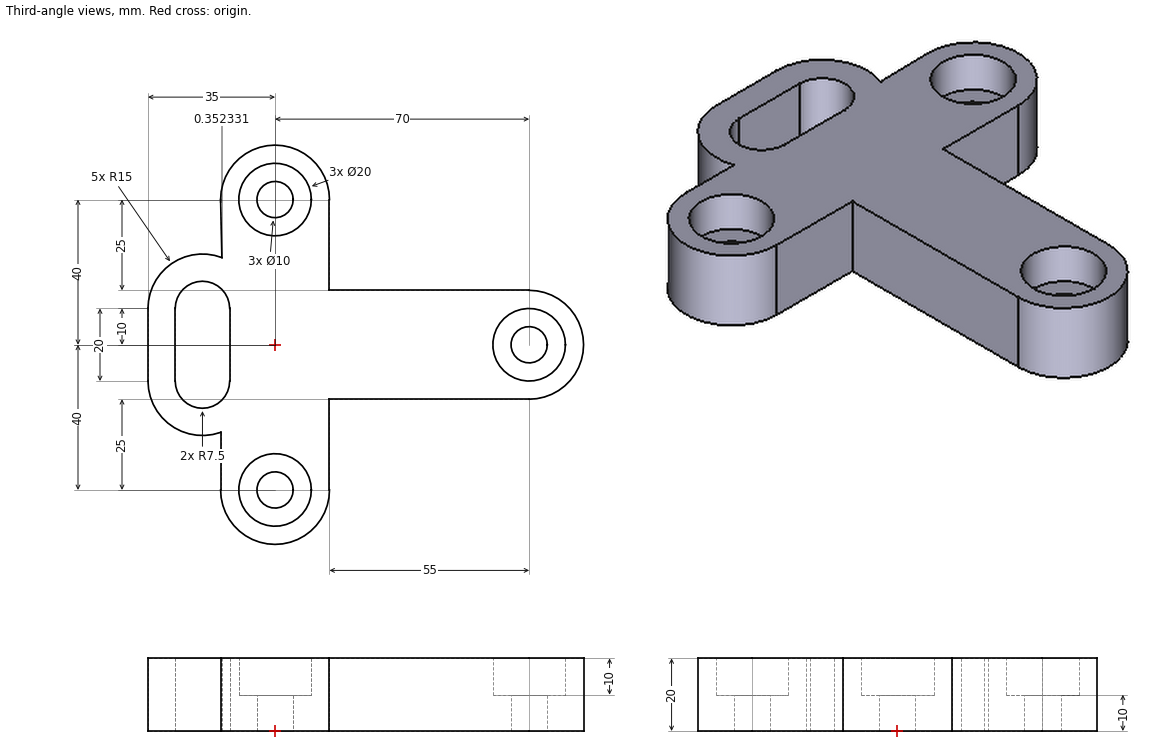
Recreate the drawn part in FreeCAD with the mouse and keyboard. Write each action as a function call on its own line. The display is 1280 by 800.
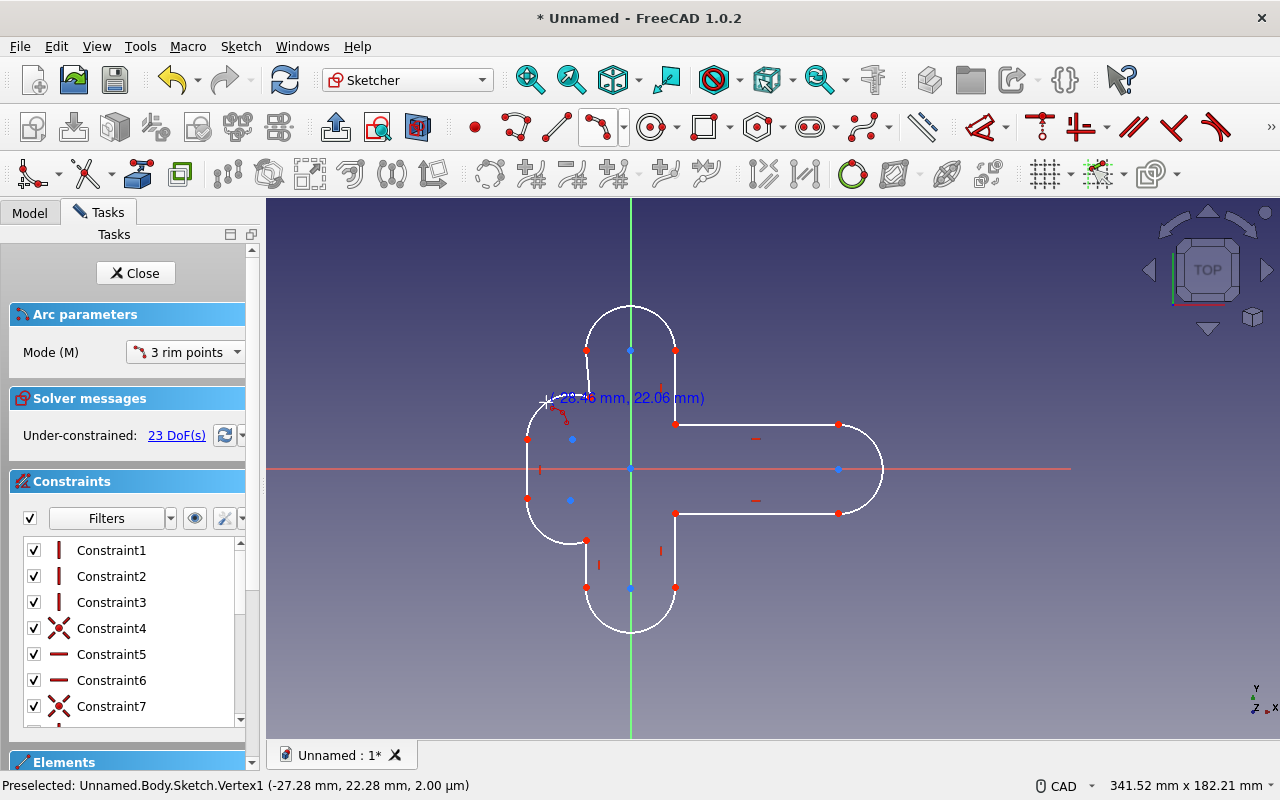
click(810, 128)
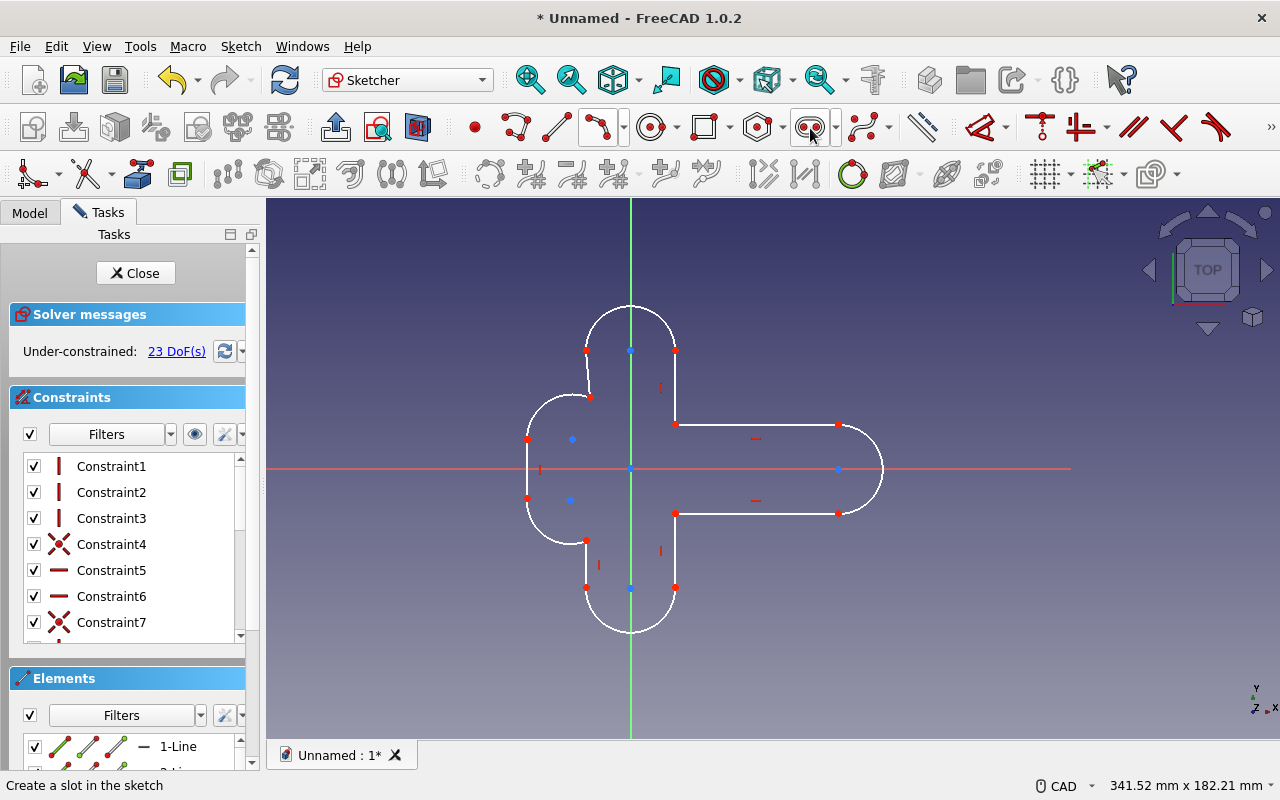
click(571, 498)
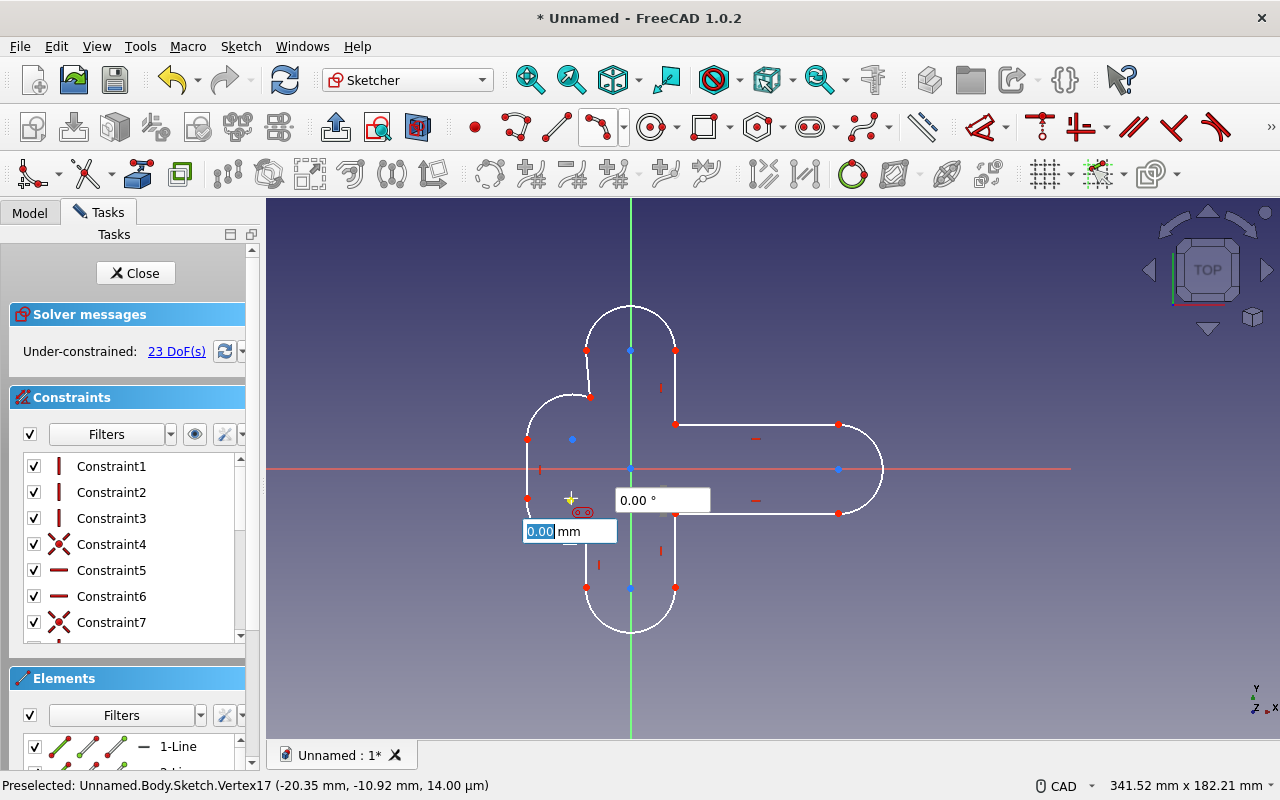
click(571, 439)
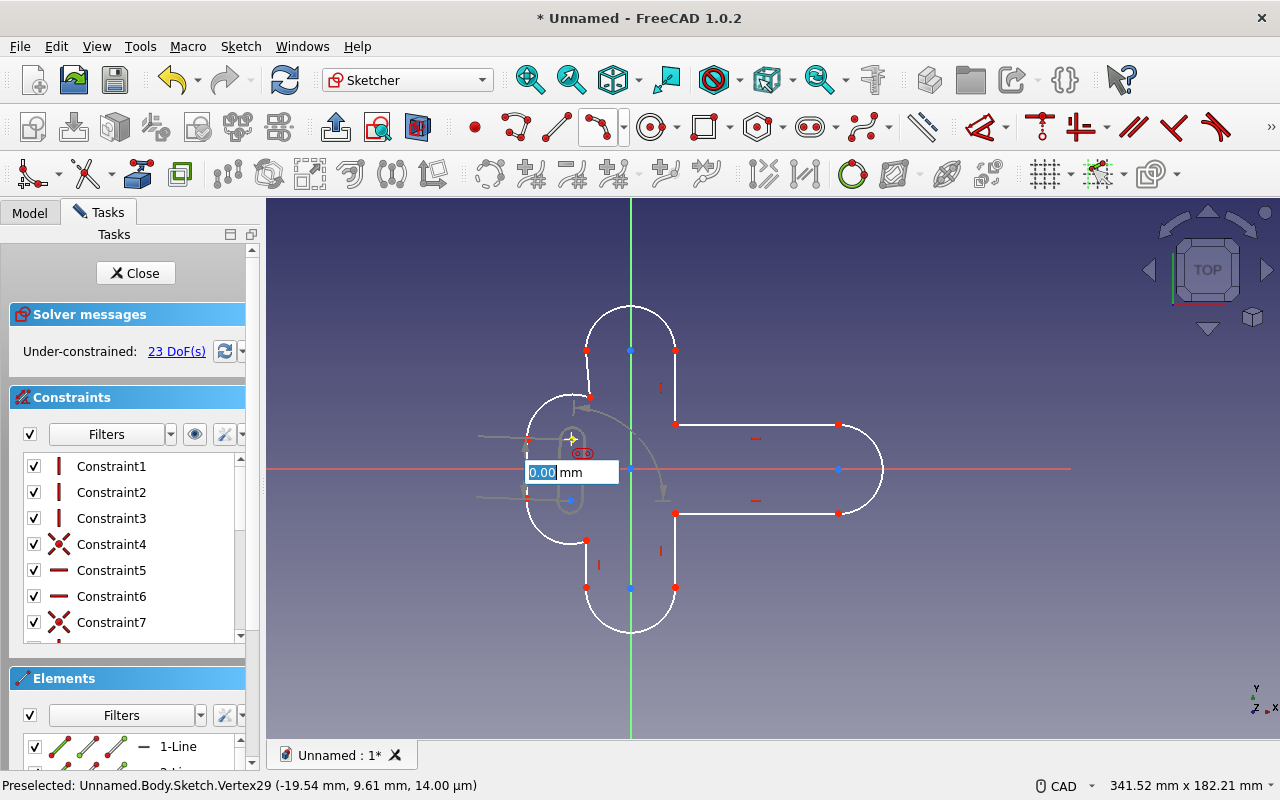
scroll(549, 477, up, 3)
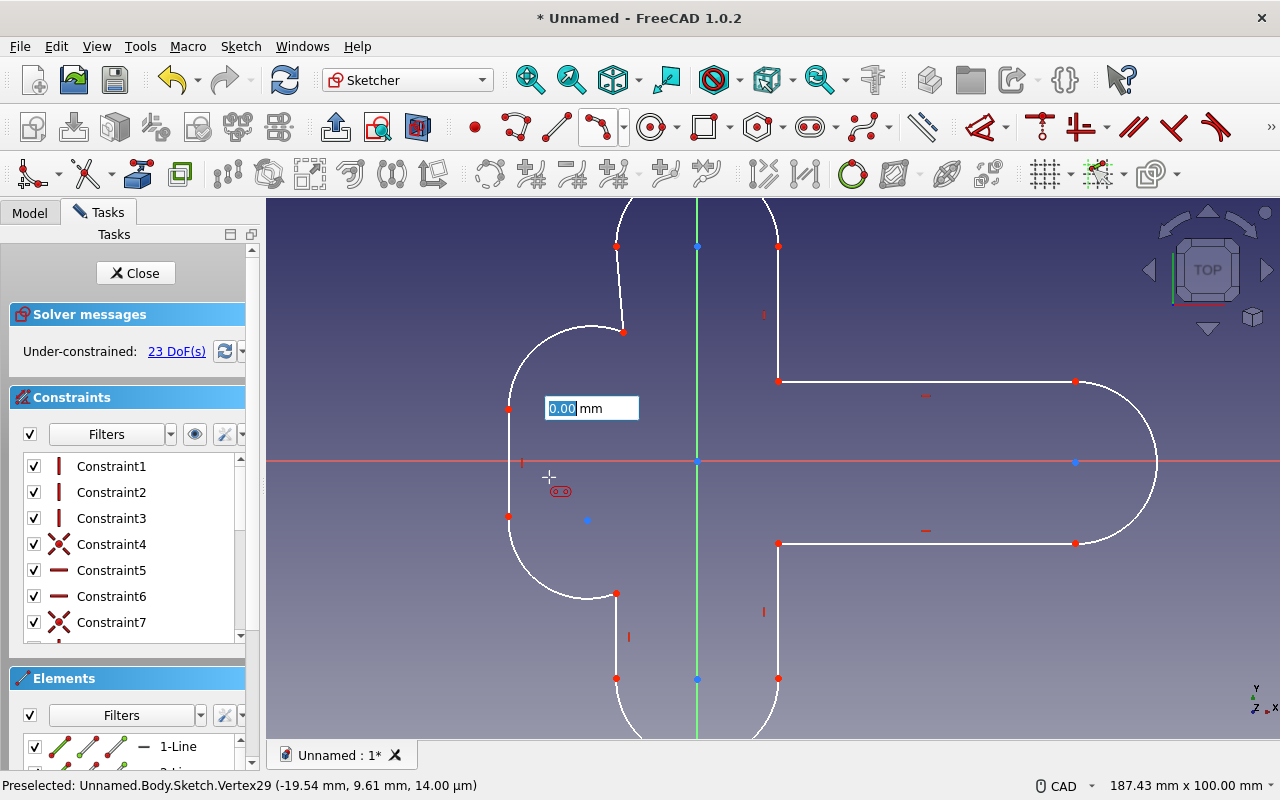
click(549, 477)
key(Escape)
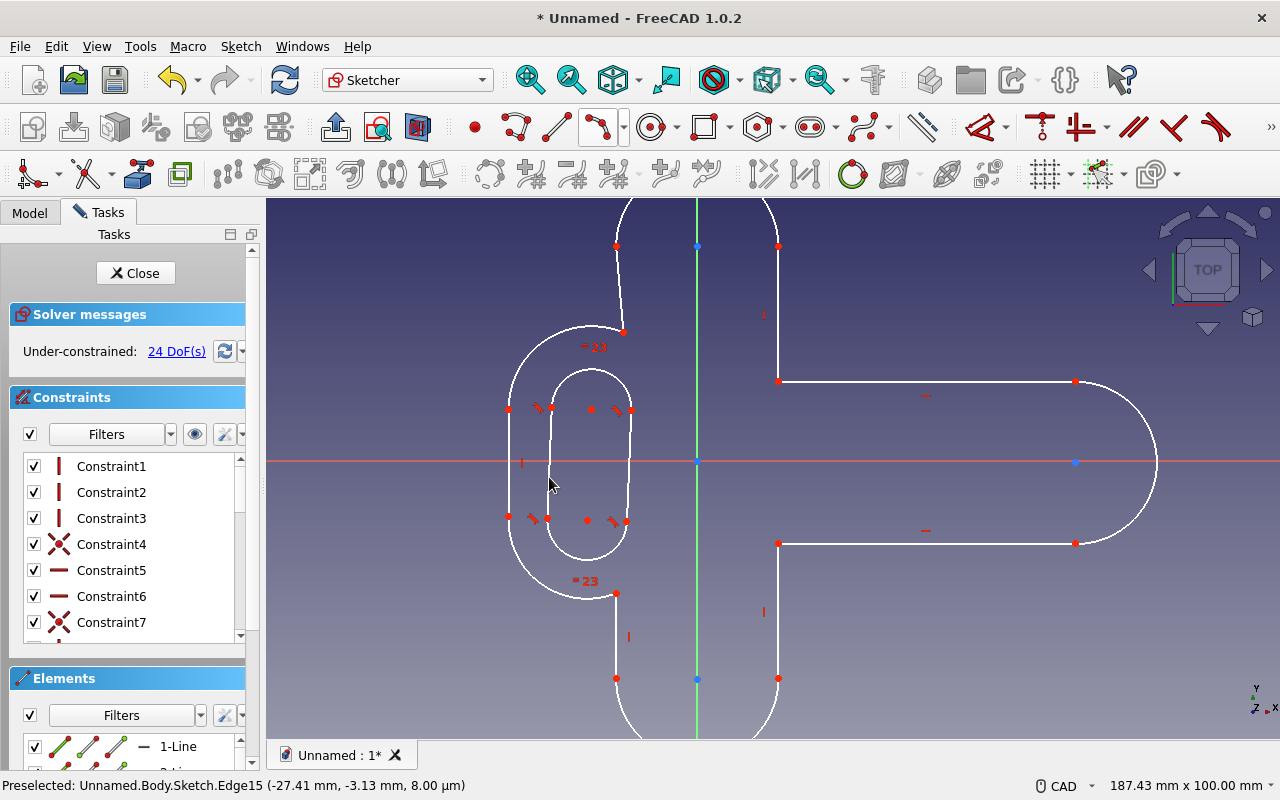
click(509, 441)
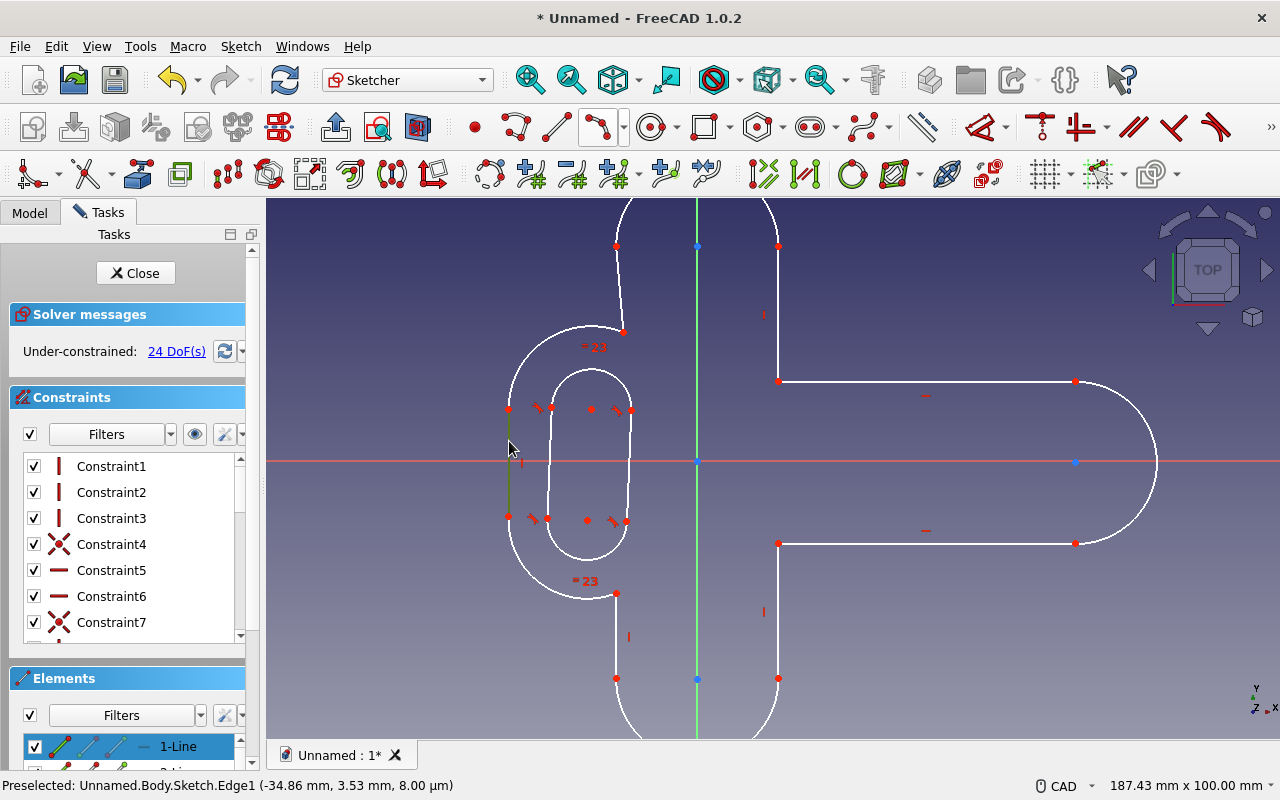
click(520, 561)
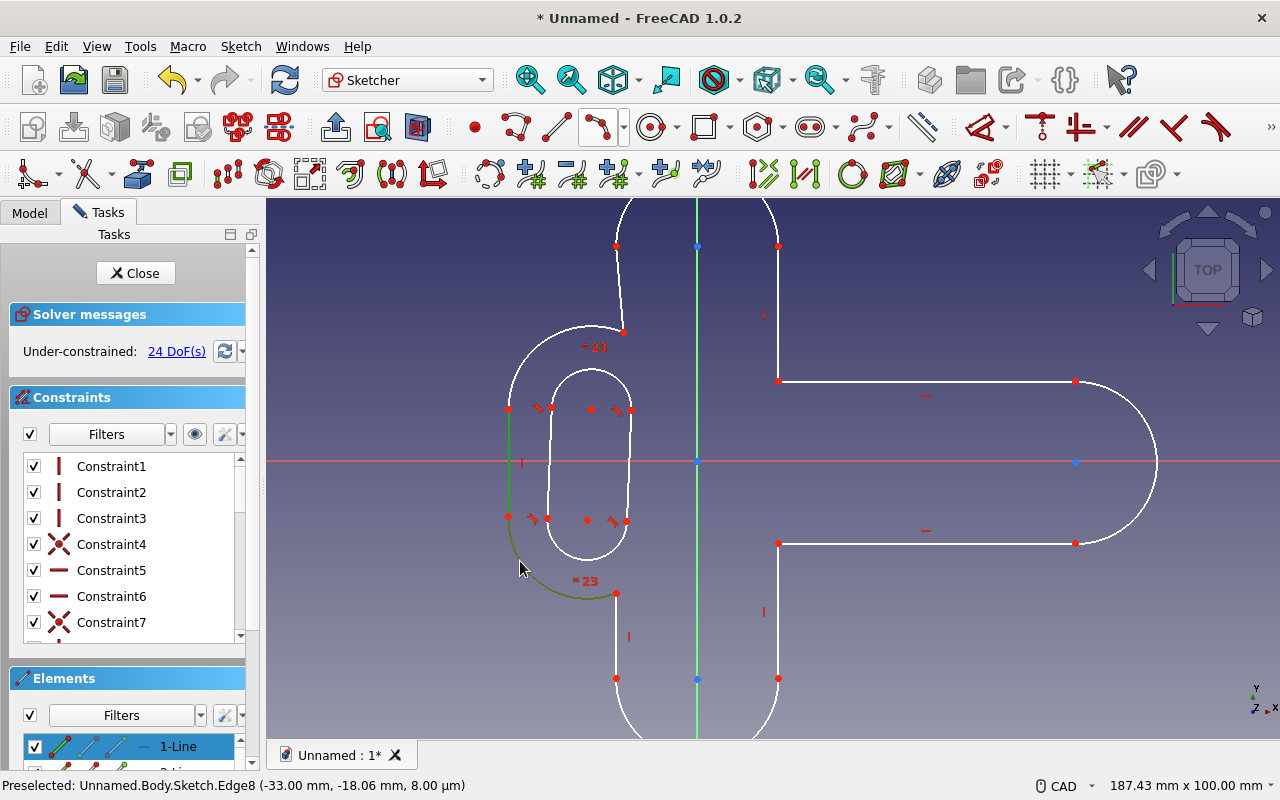
key(t)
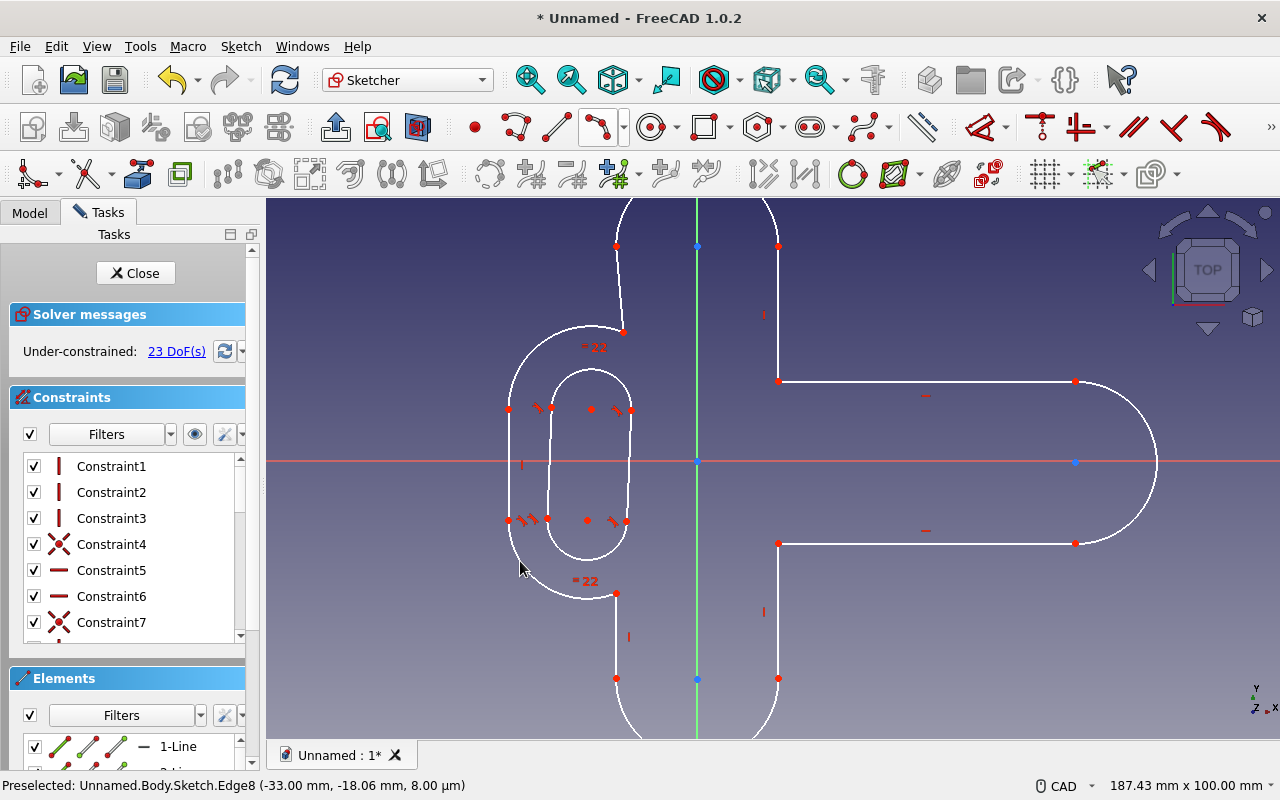
click(509, 442)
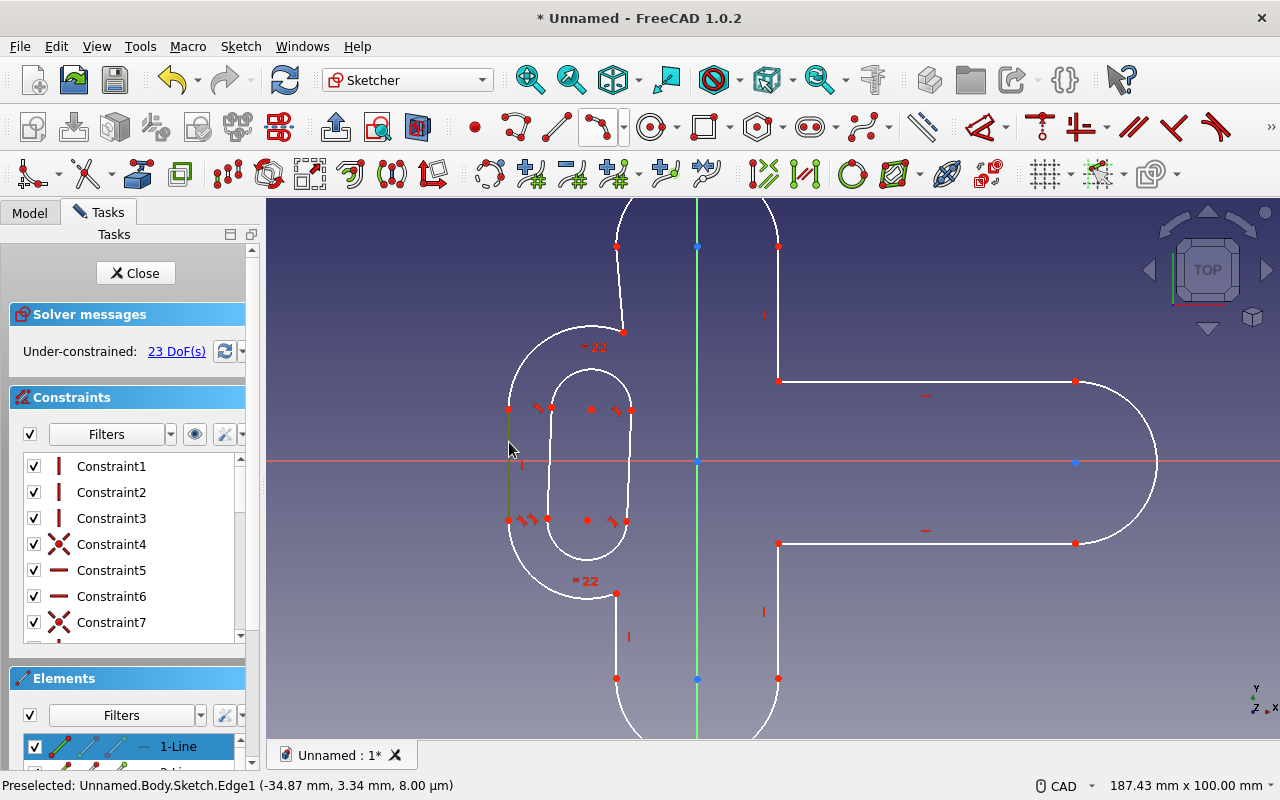
click(576, 328)